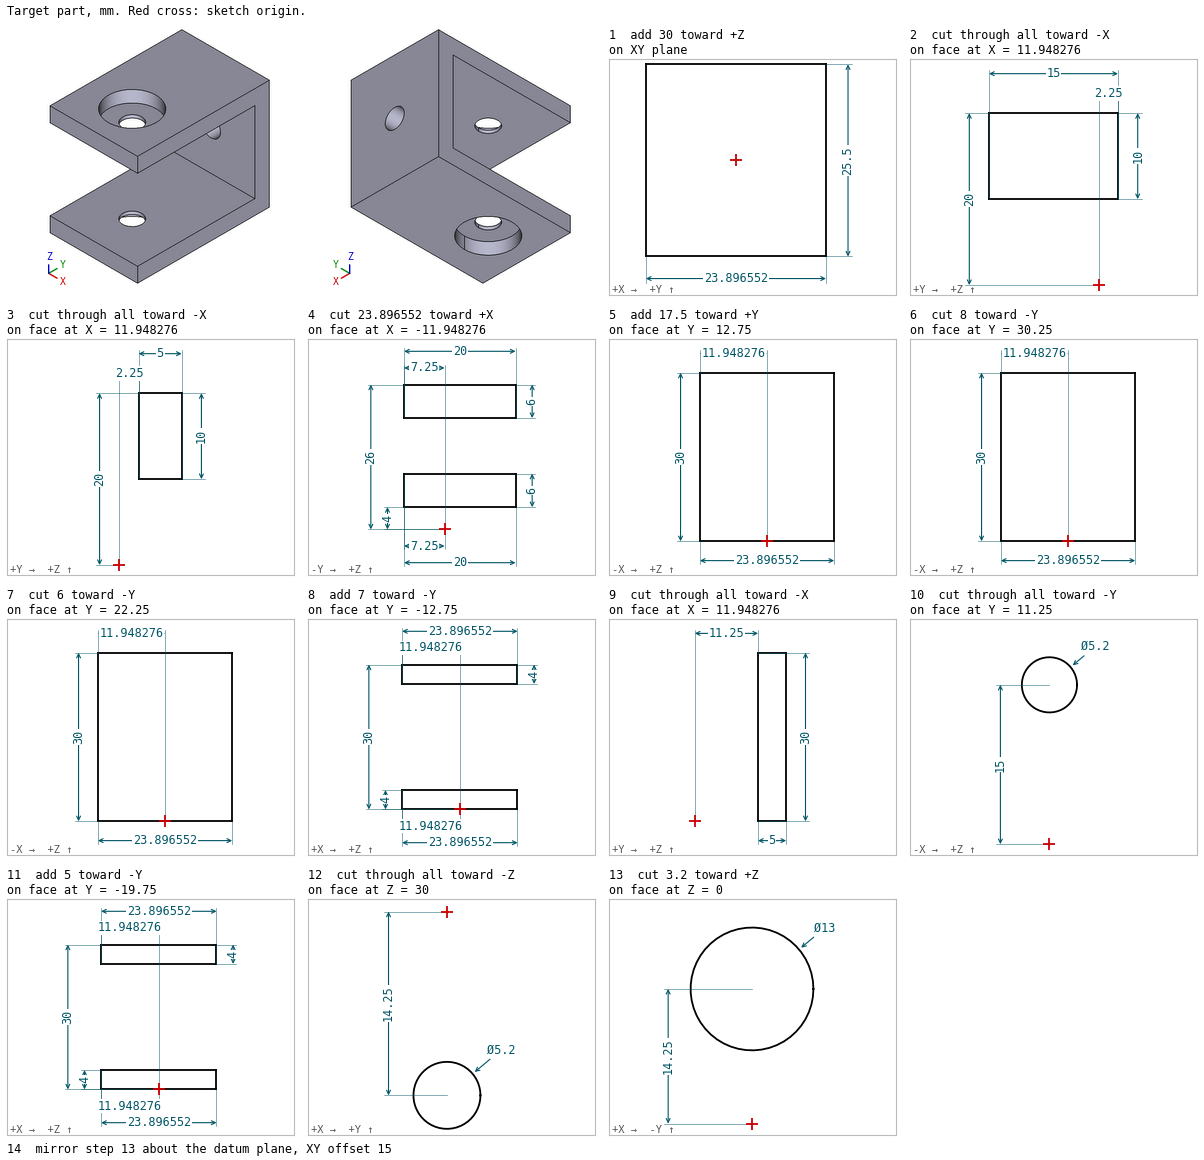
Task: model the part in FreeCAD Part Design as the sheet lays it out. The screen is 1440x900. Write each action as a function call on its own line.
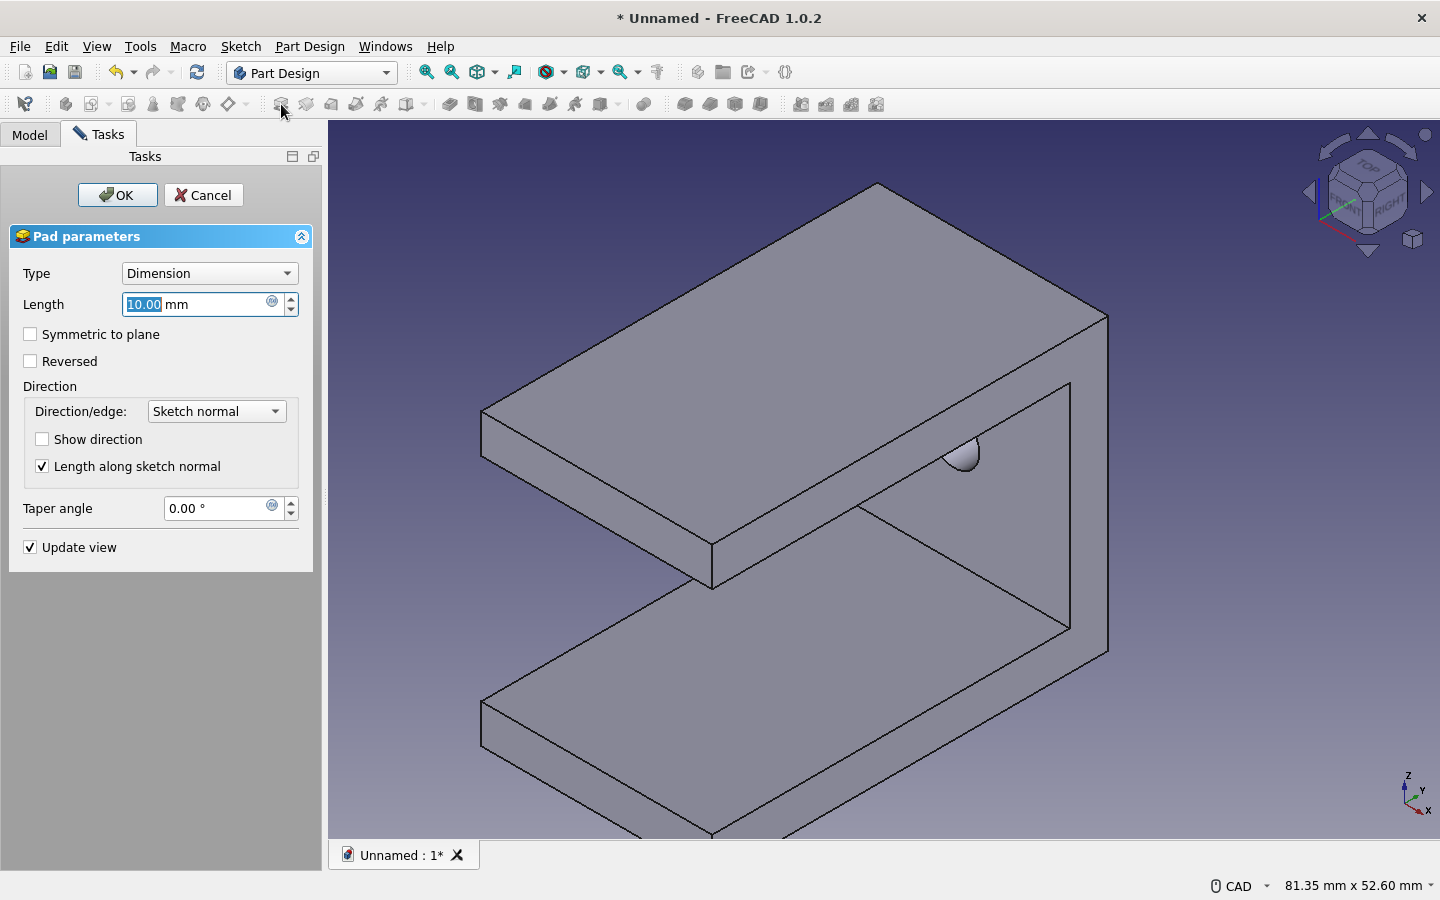
text(5)
key(Tab)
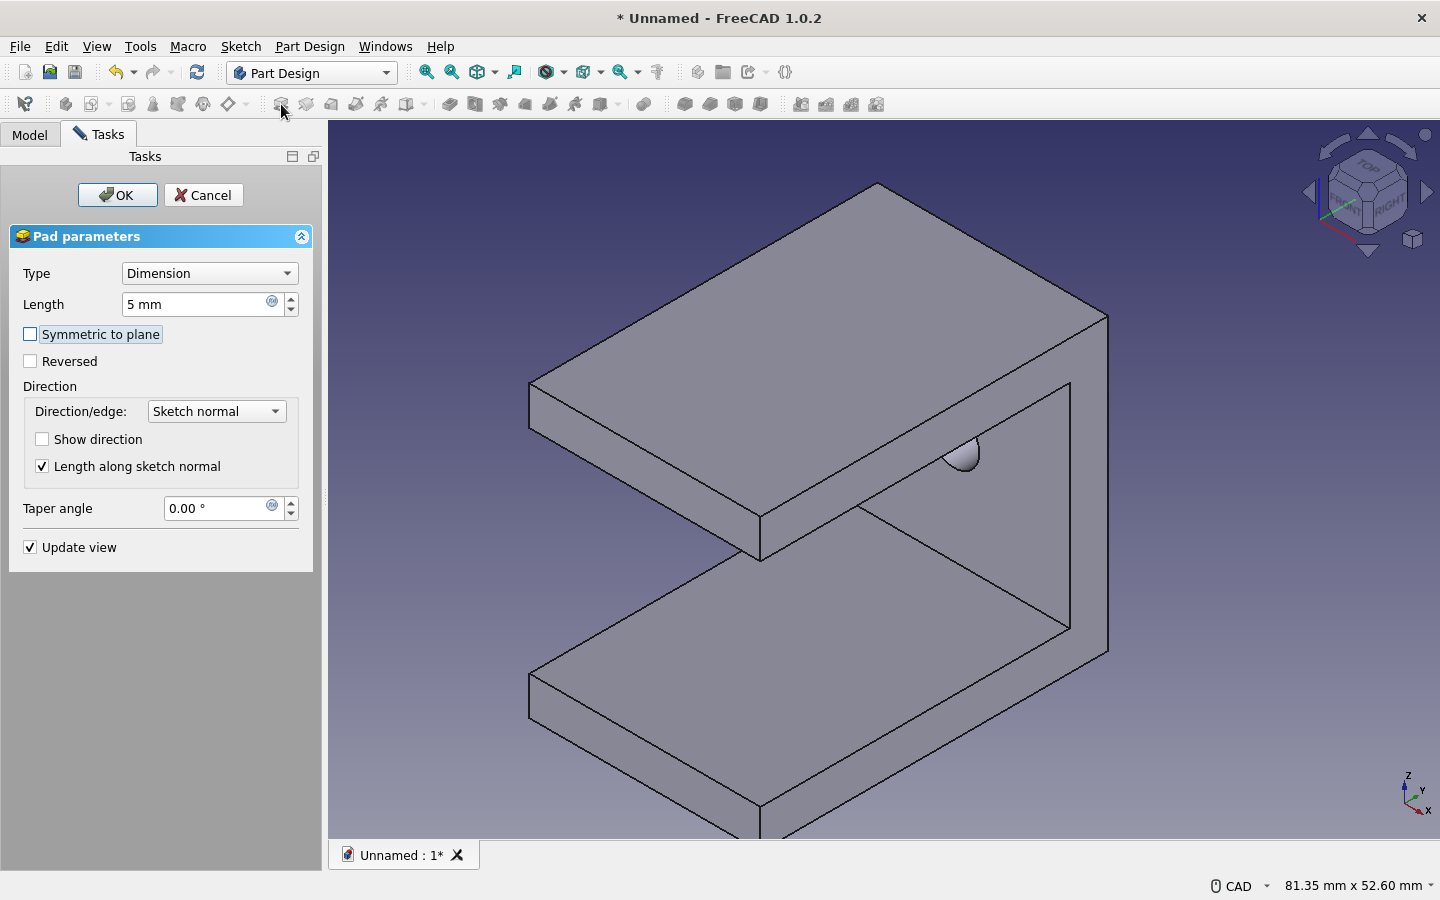
click(118, 195)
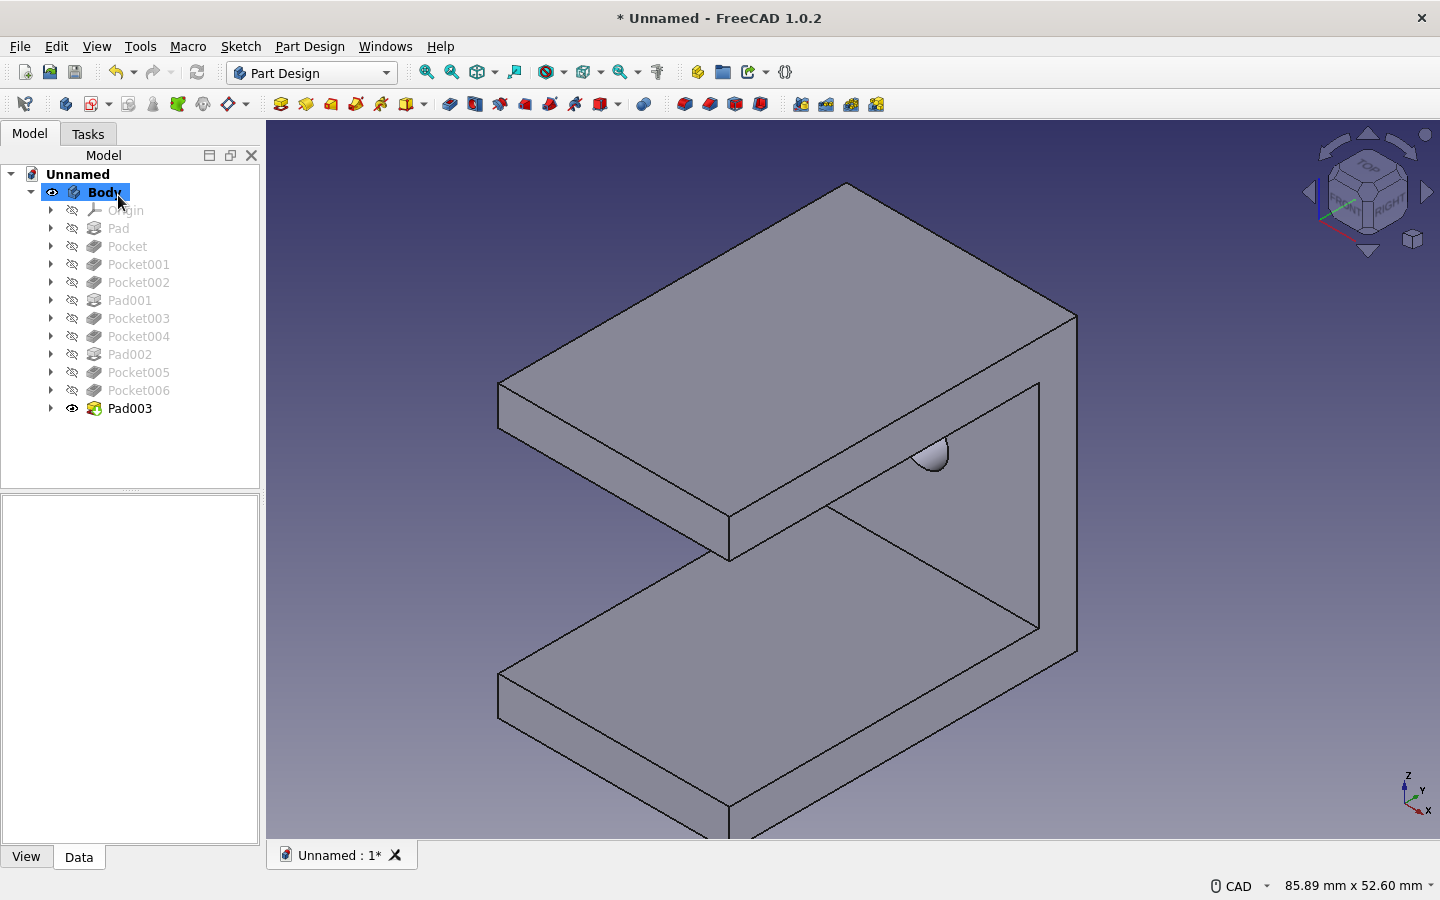
click(427, 72)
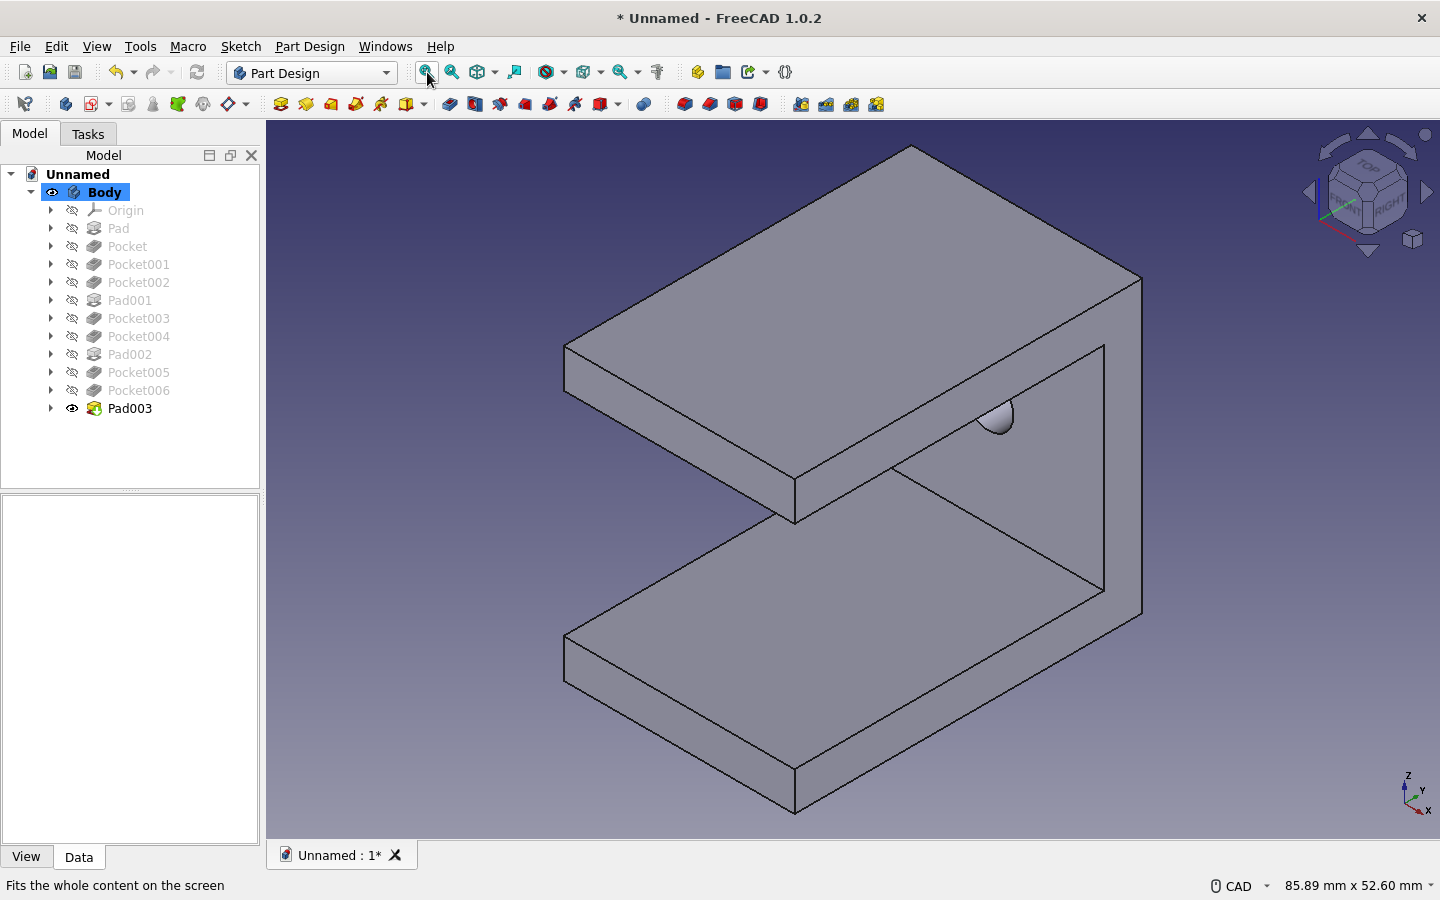
click(903, 282)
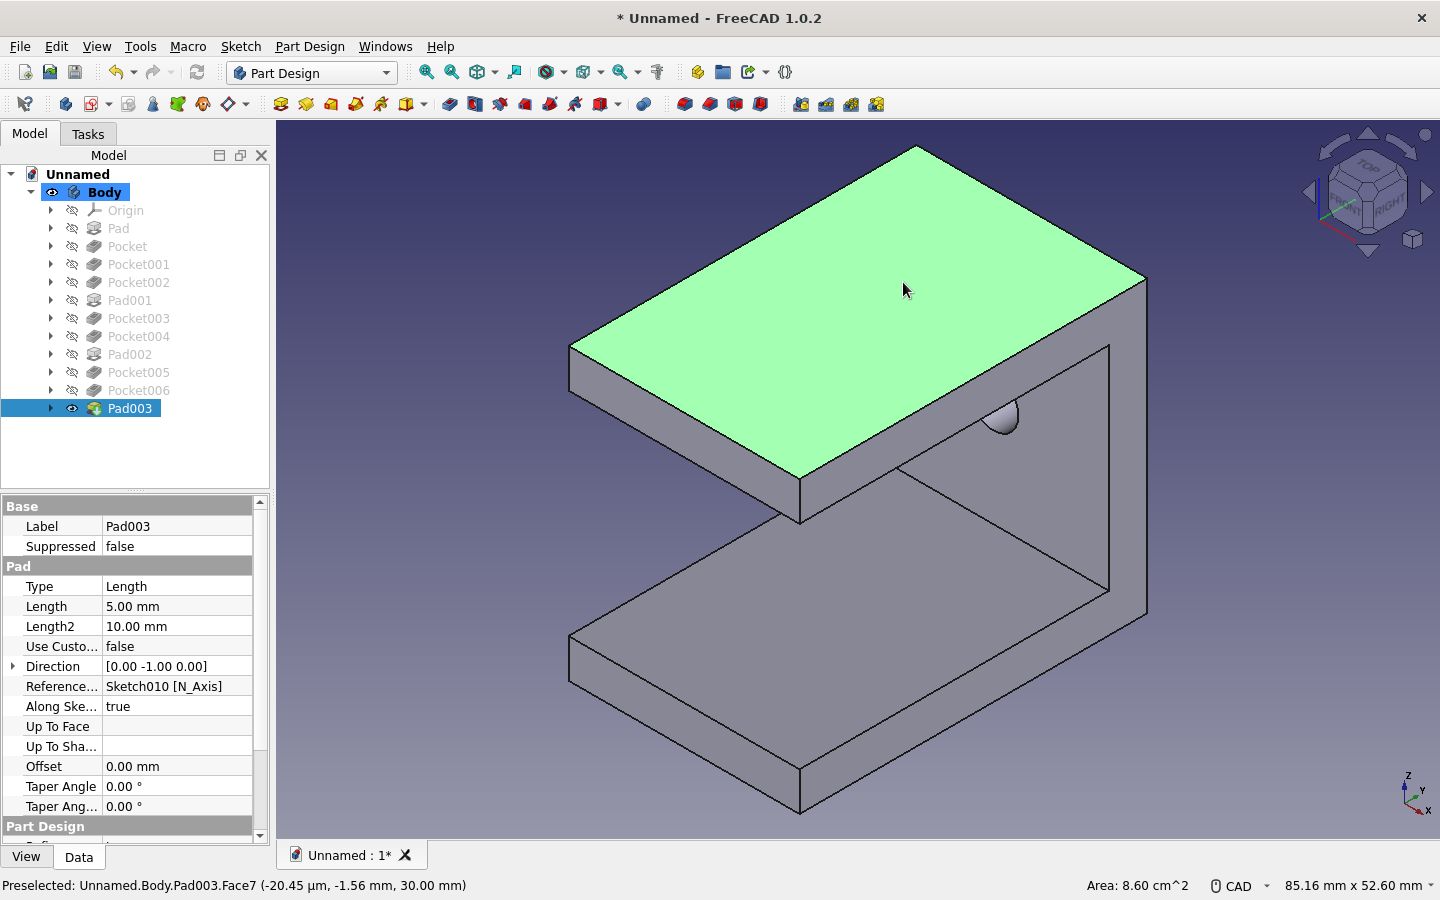
click(90, 104)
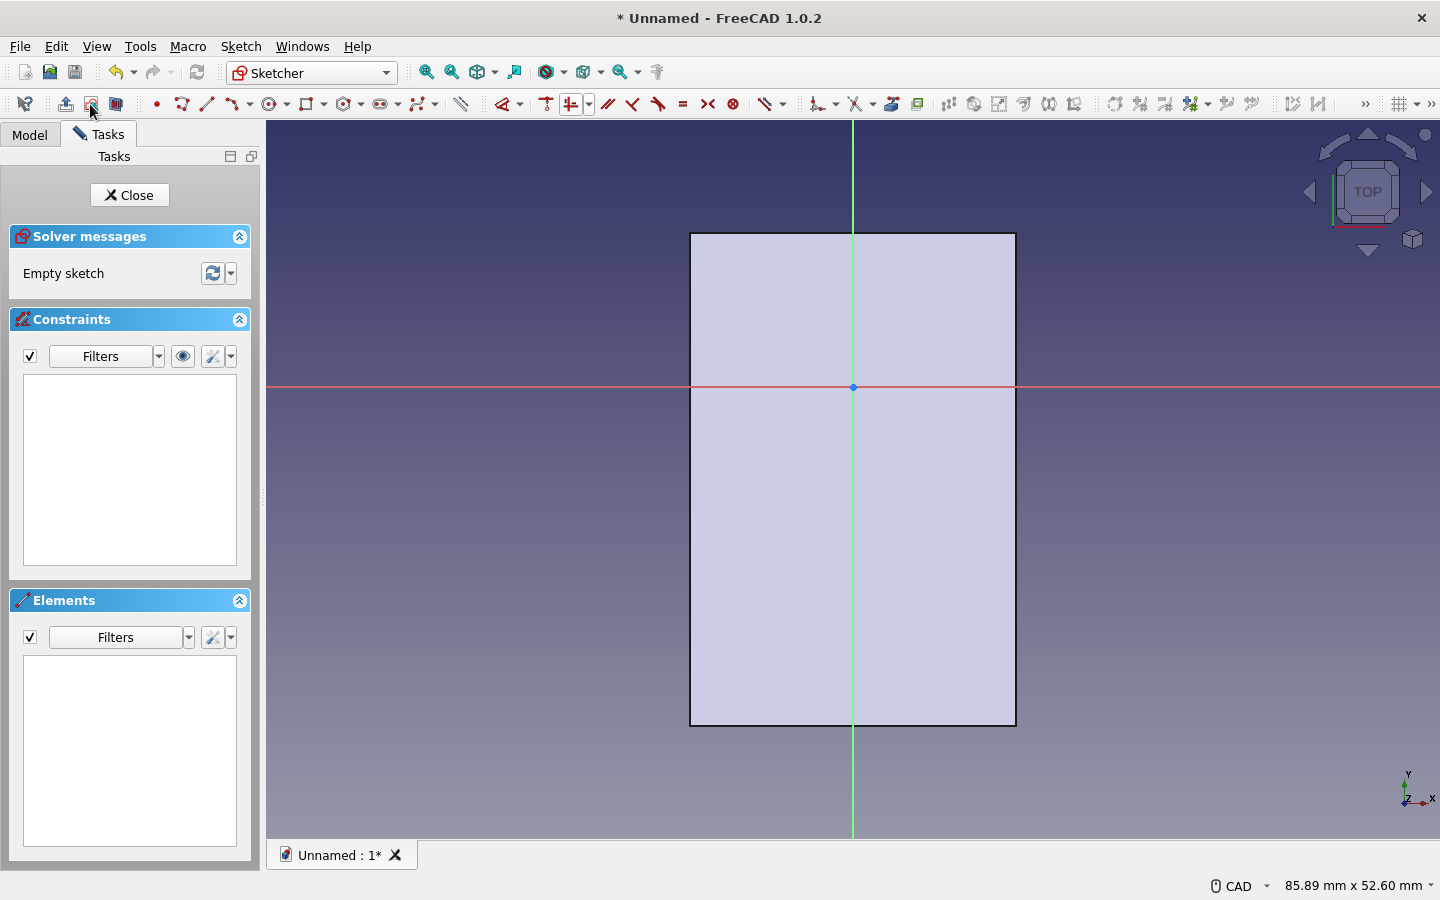
scroll(867, 602, up, 9)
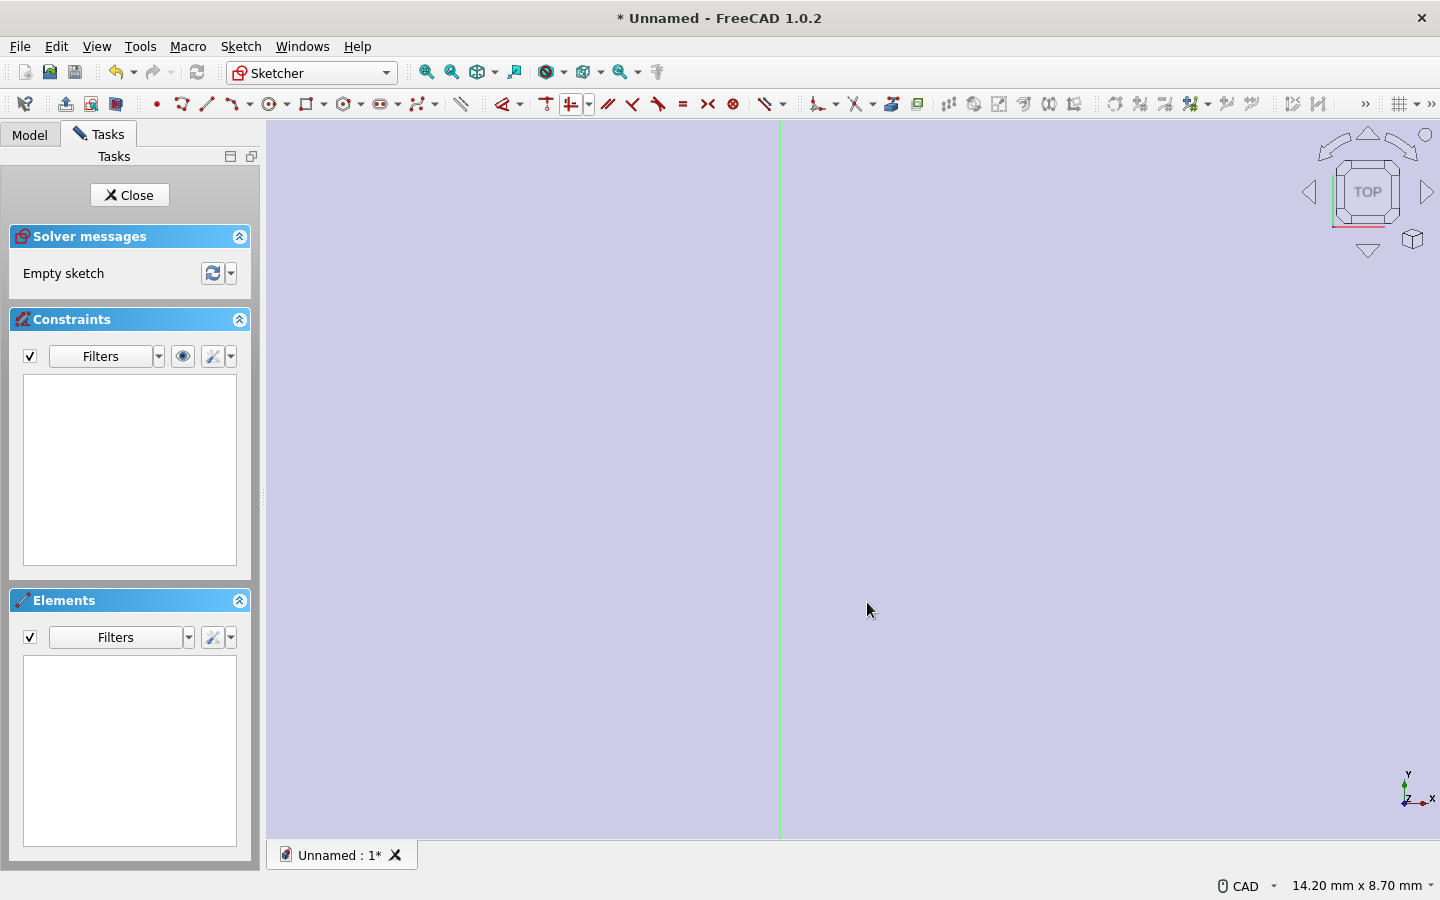
key(g)
key(c)